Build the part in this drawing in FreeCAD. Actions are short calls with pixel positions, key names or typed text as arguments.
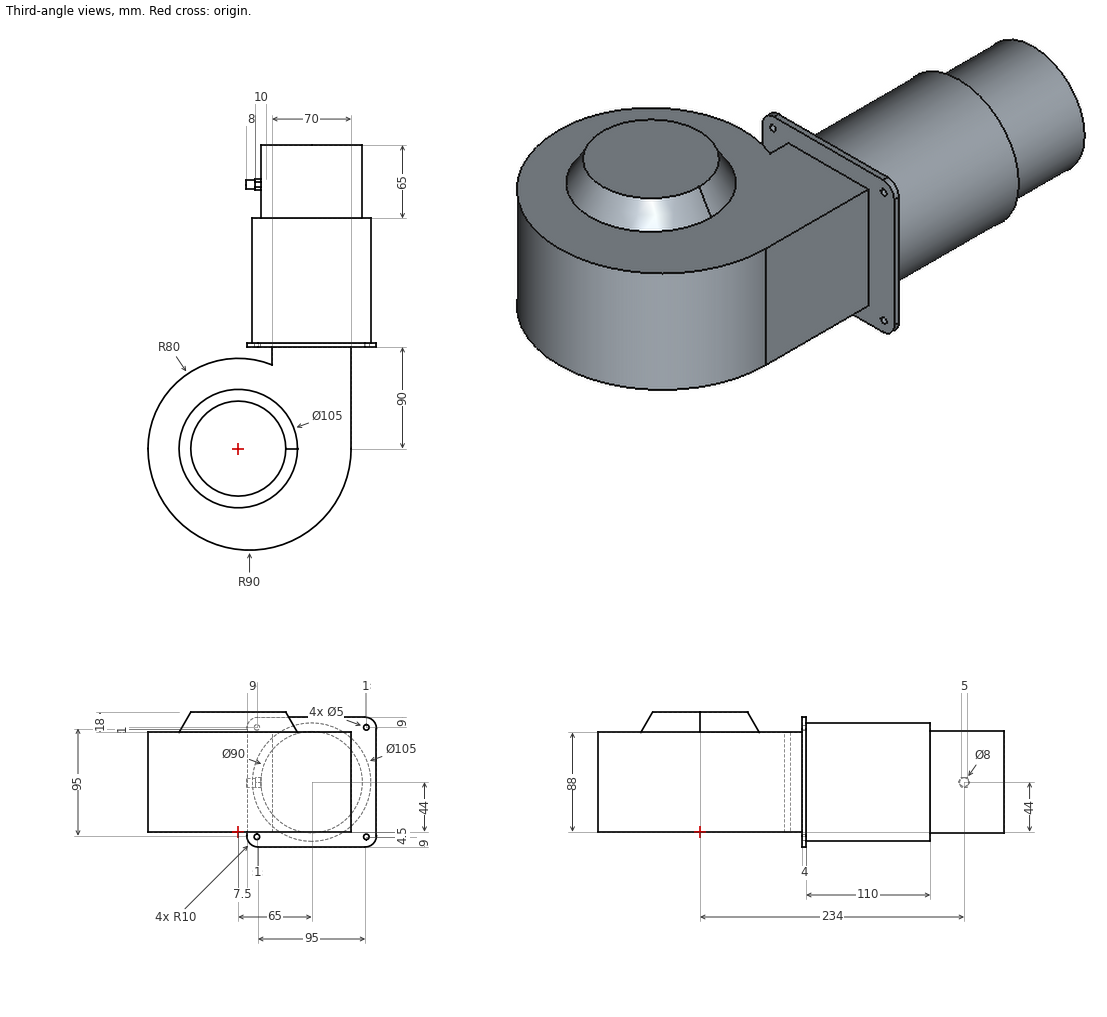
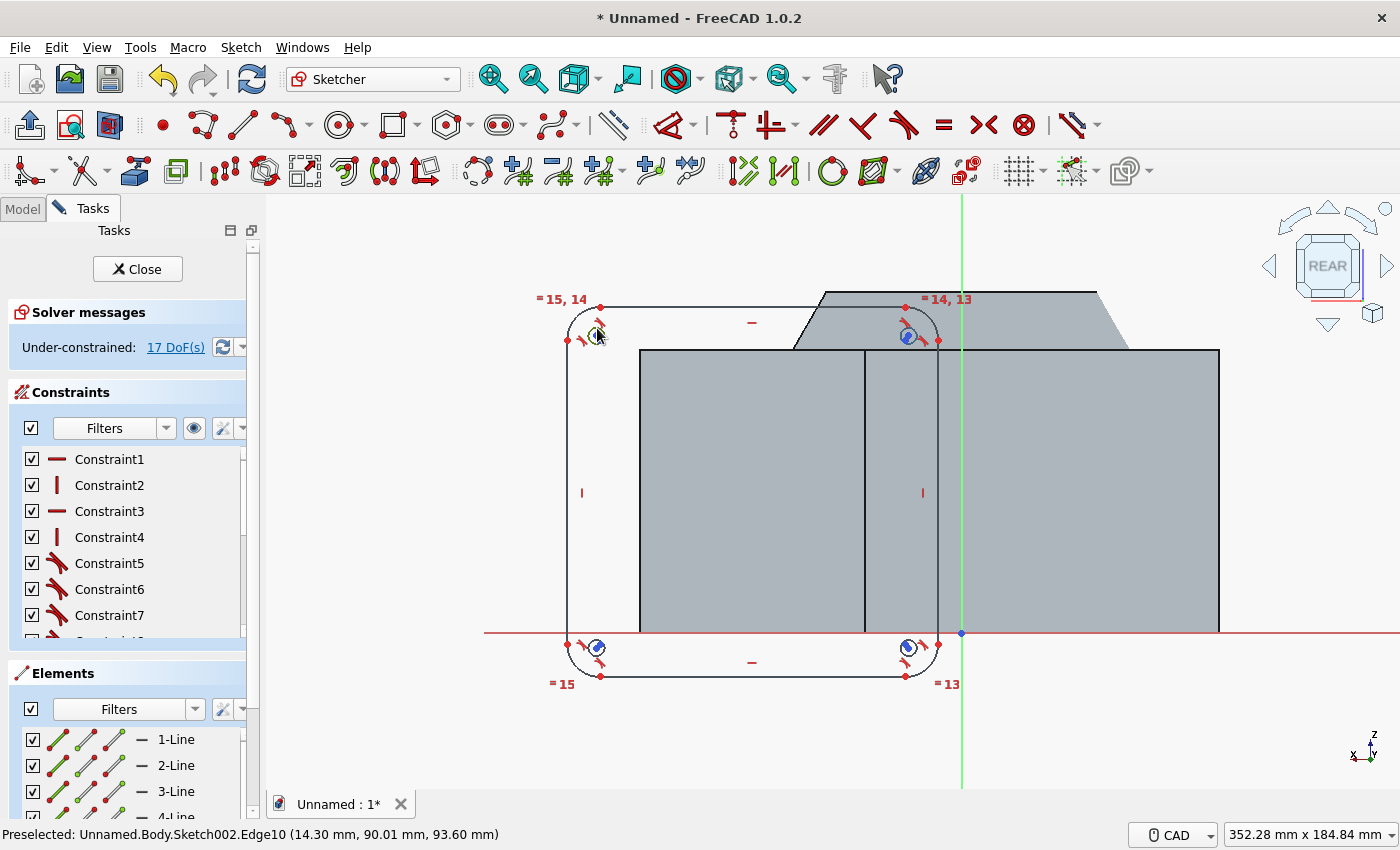
scroll(602, 642, up, 3)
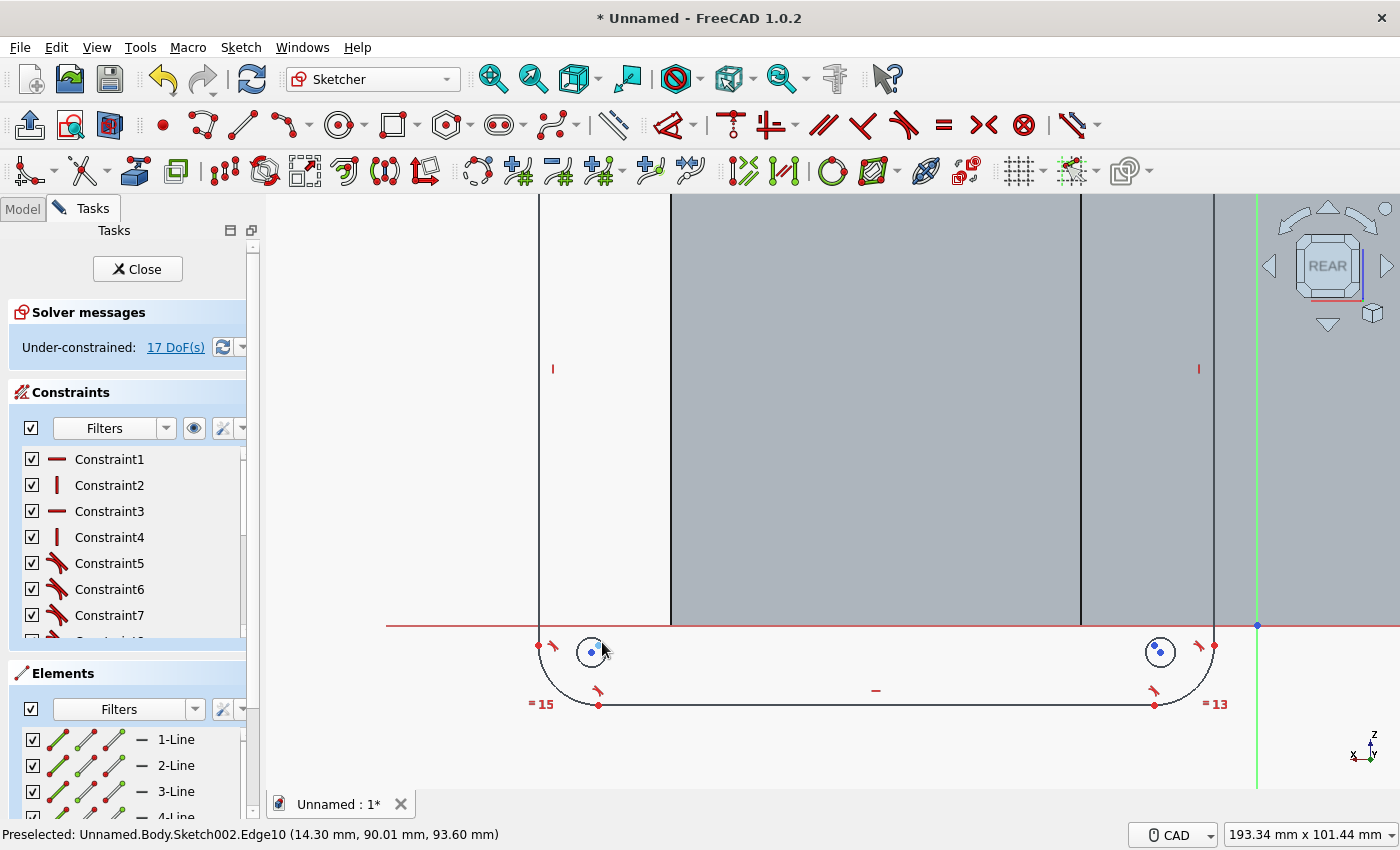
click(581, 642)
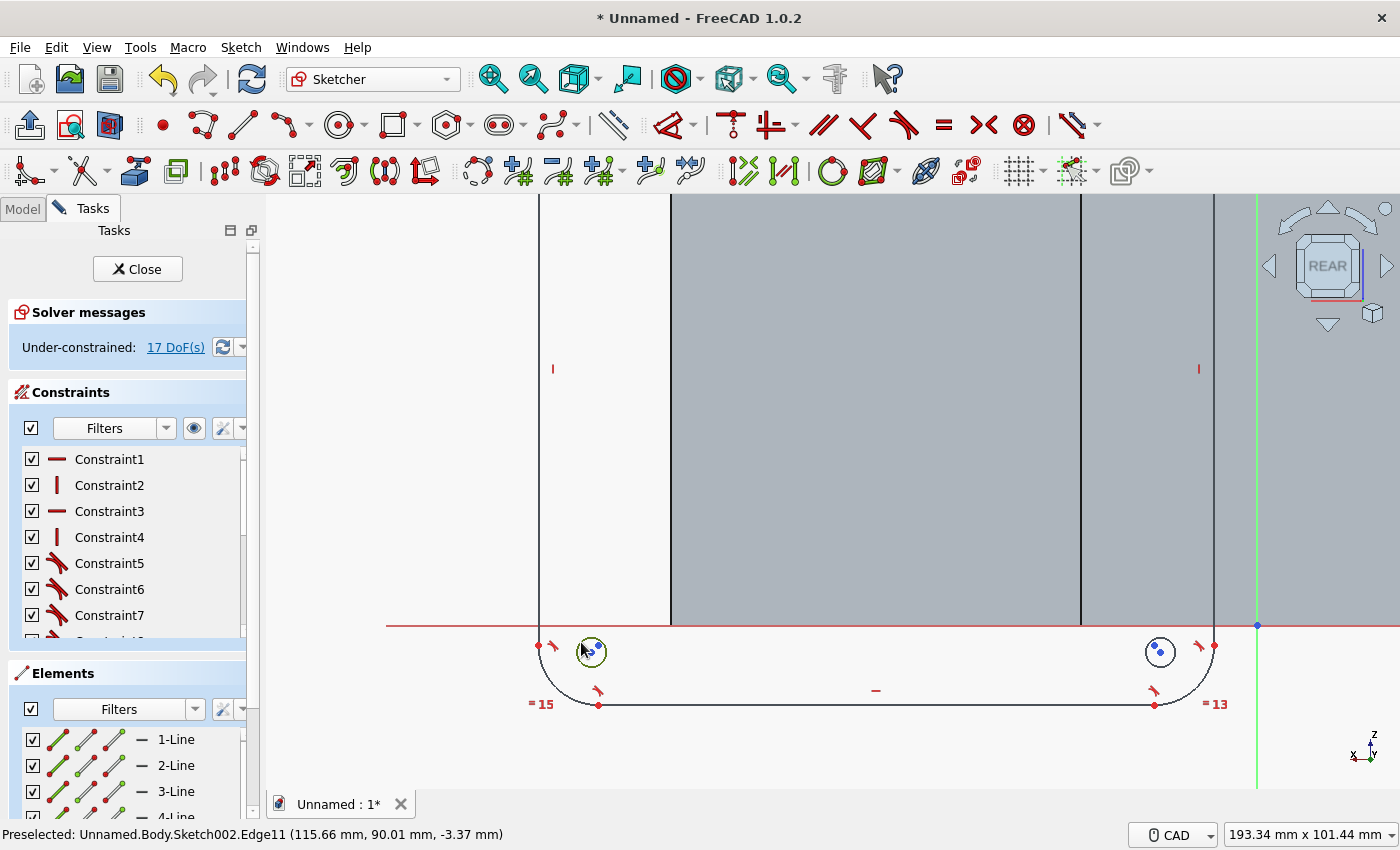
click(1171, 642)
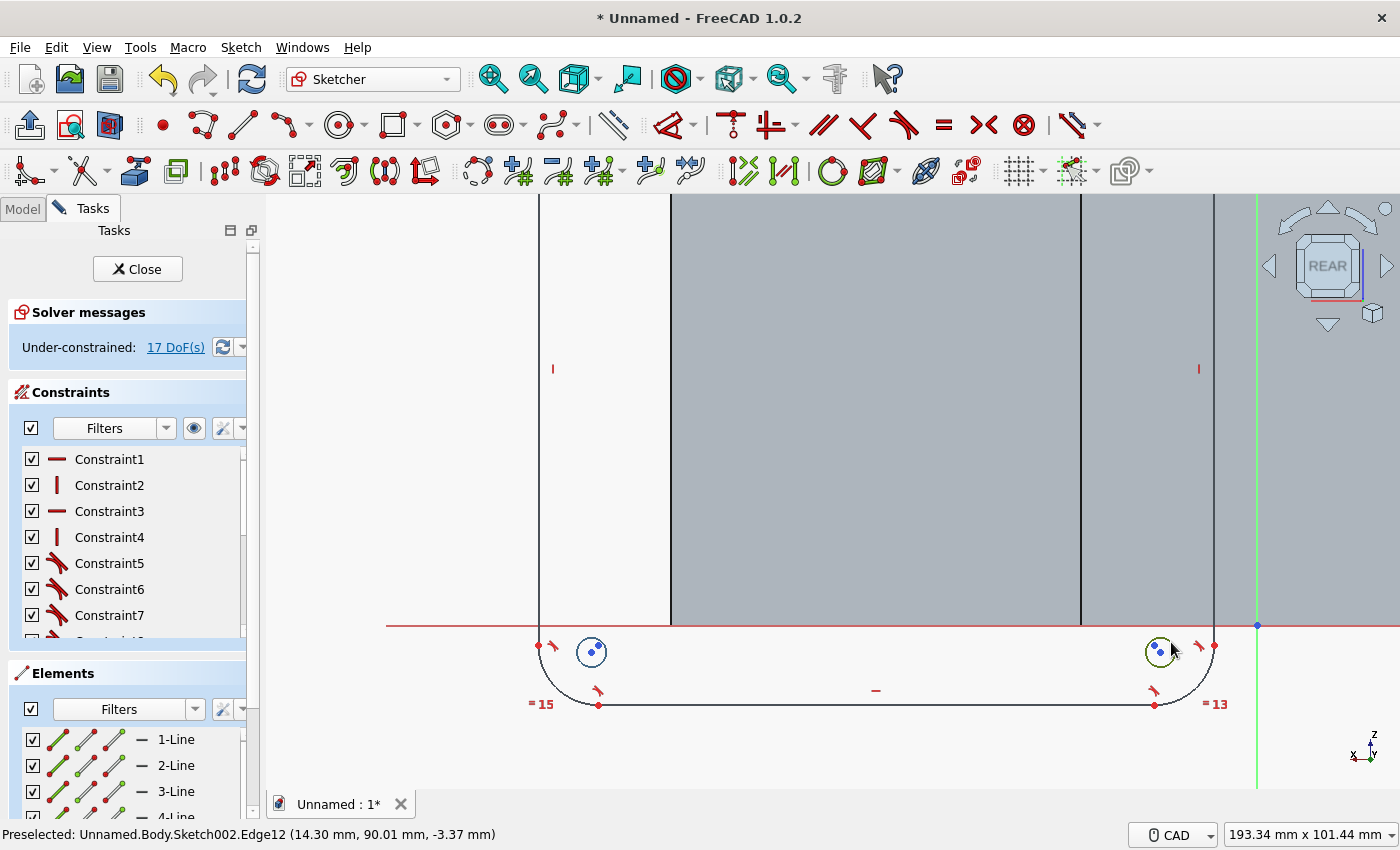
click(944, 126)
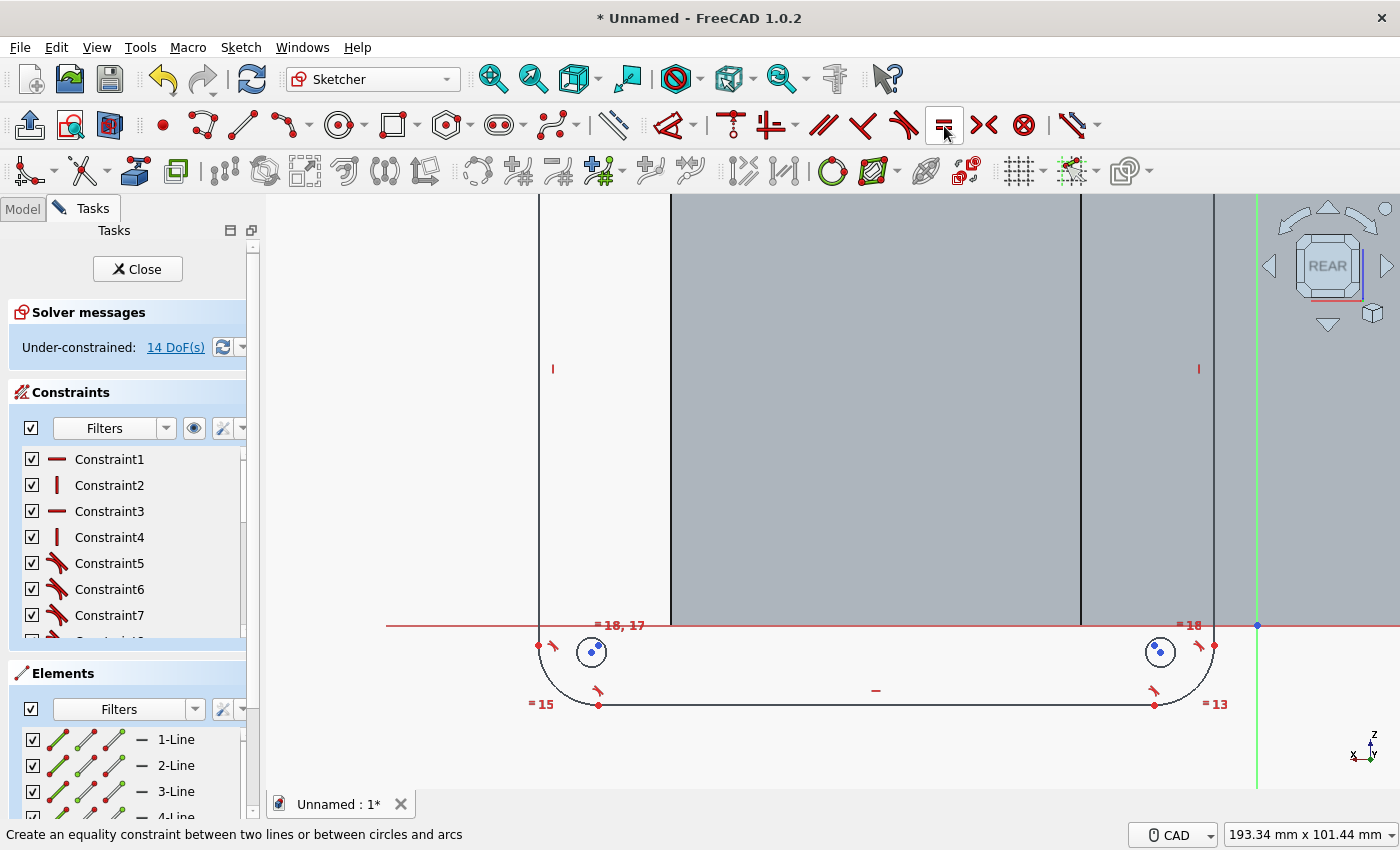
click(668, 126)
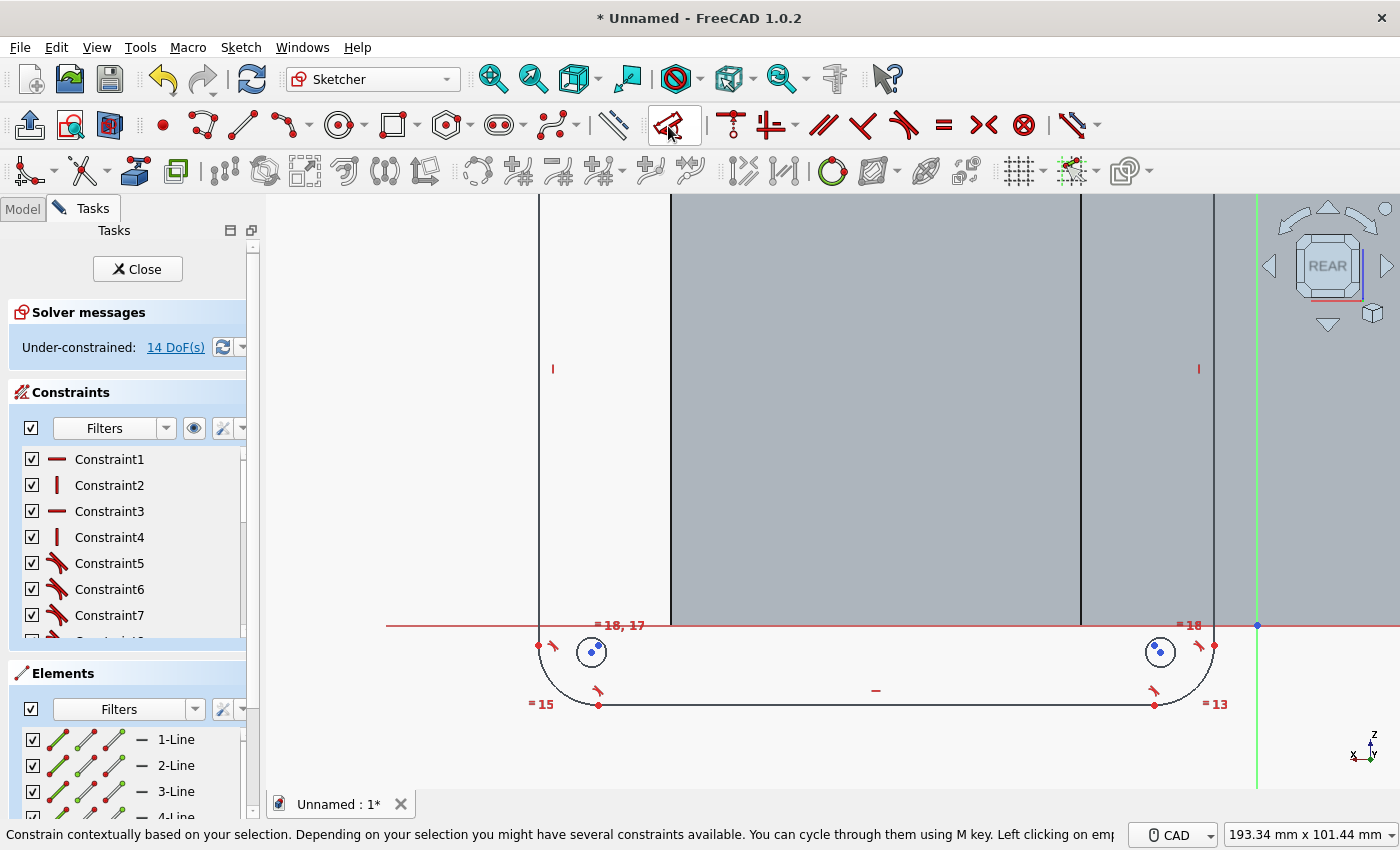
click(1181, 699)
click(1195, 728)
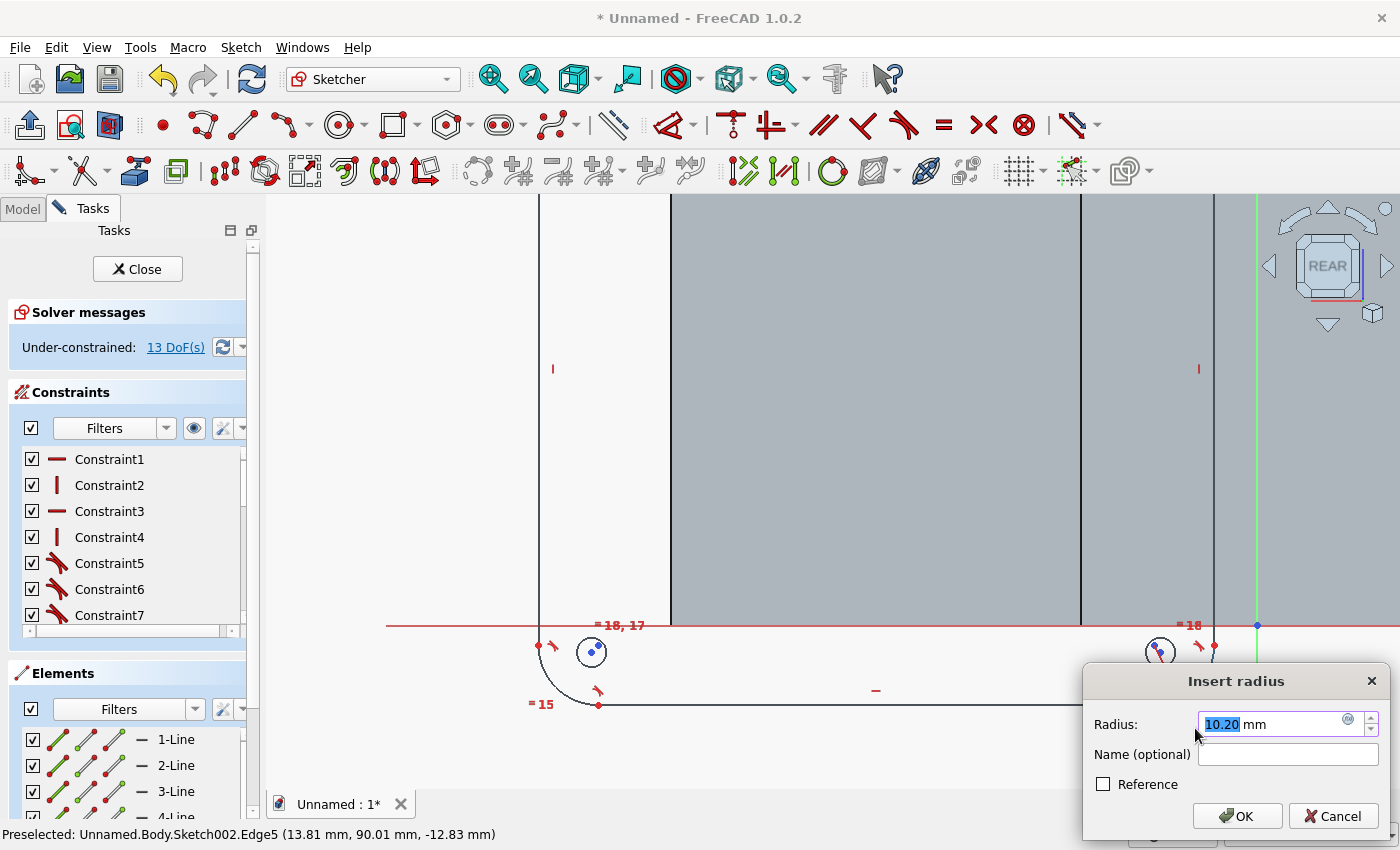
text(10)
key(Return)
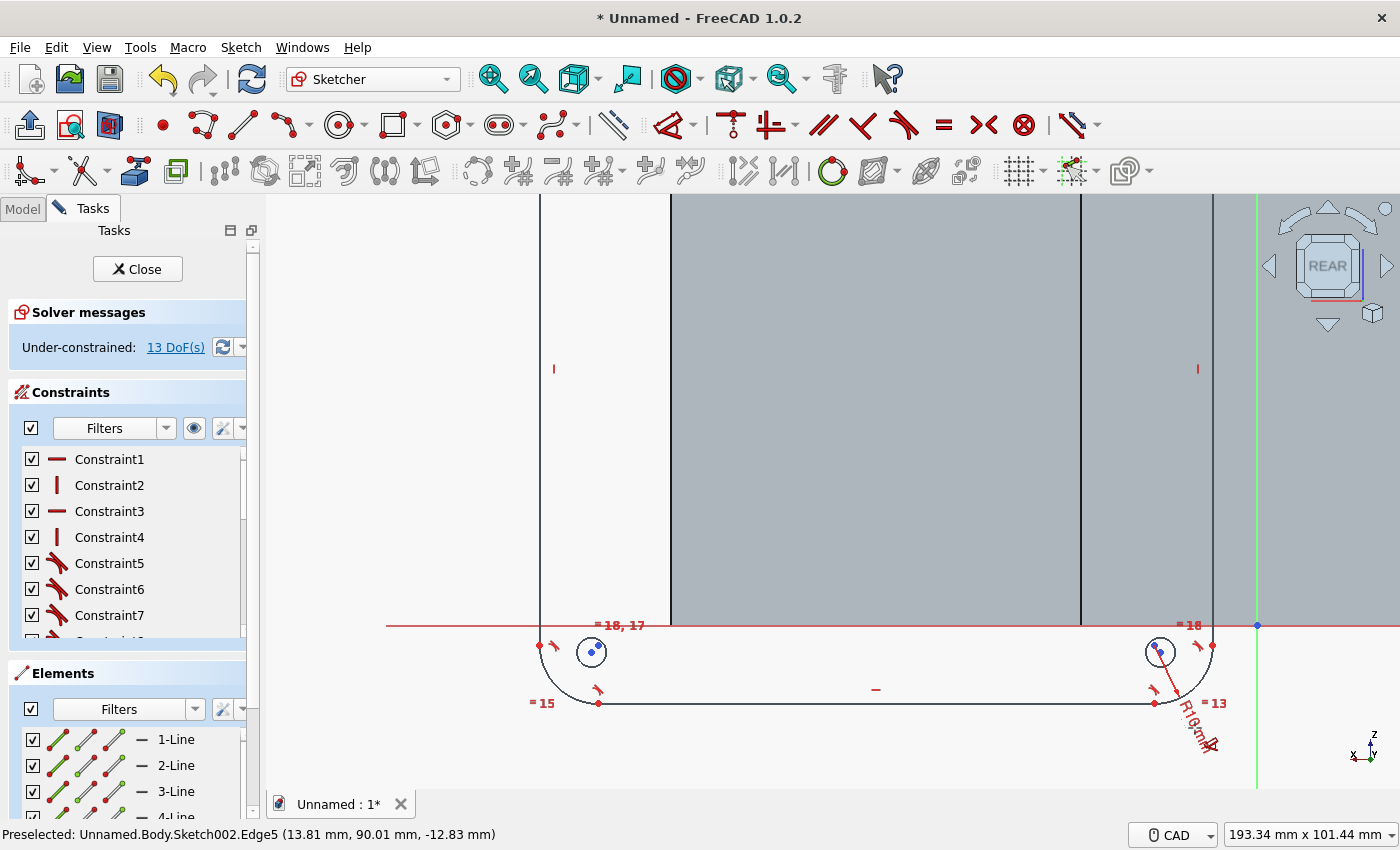
scroll(602, 642, down, 3)